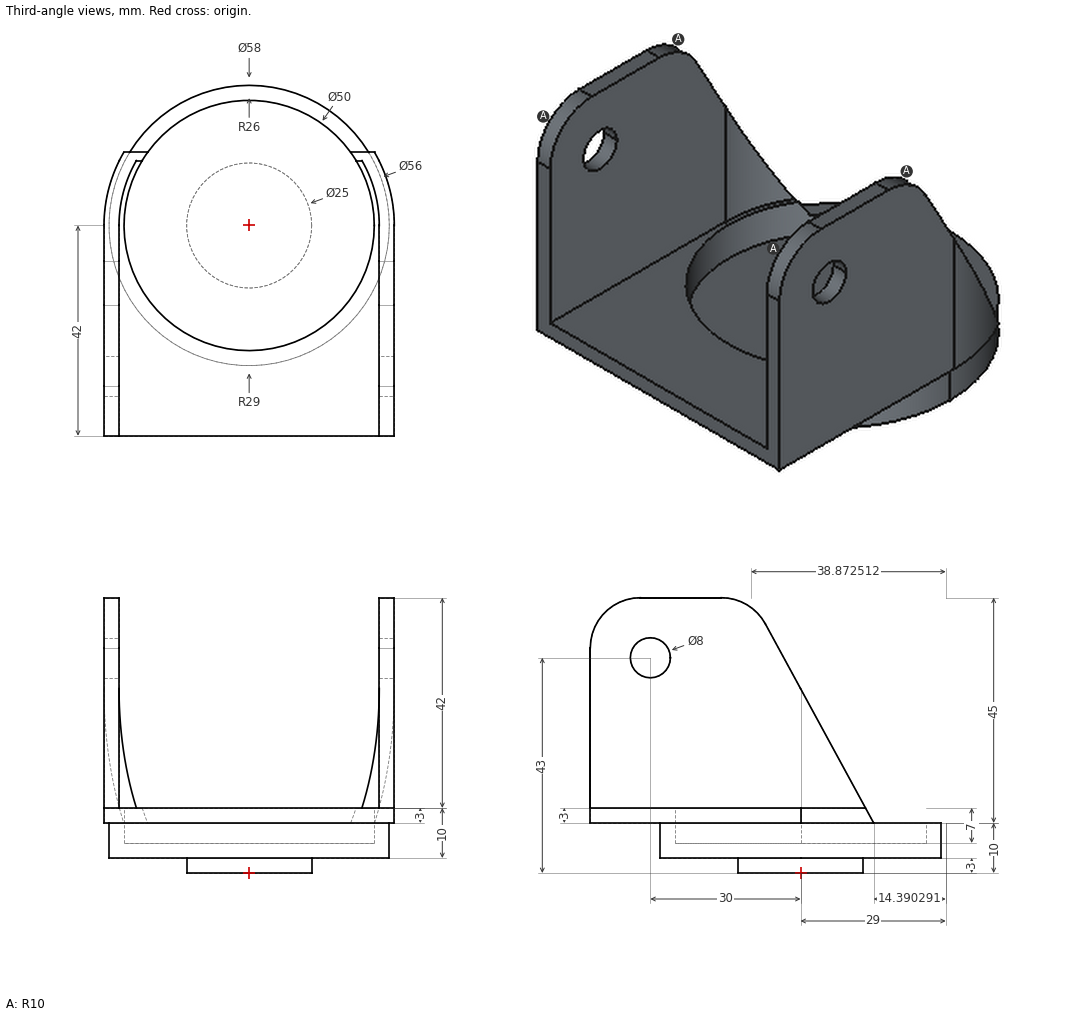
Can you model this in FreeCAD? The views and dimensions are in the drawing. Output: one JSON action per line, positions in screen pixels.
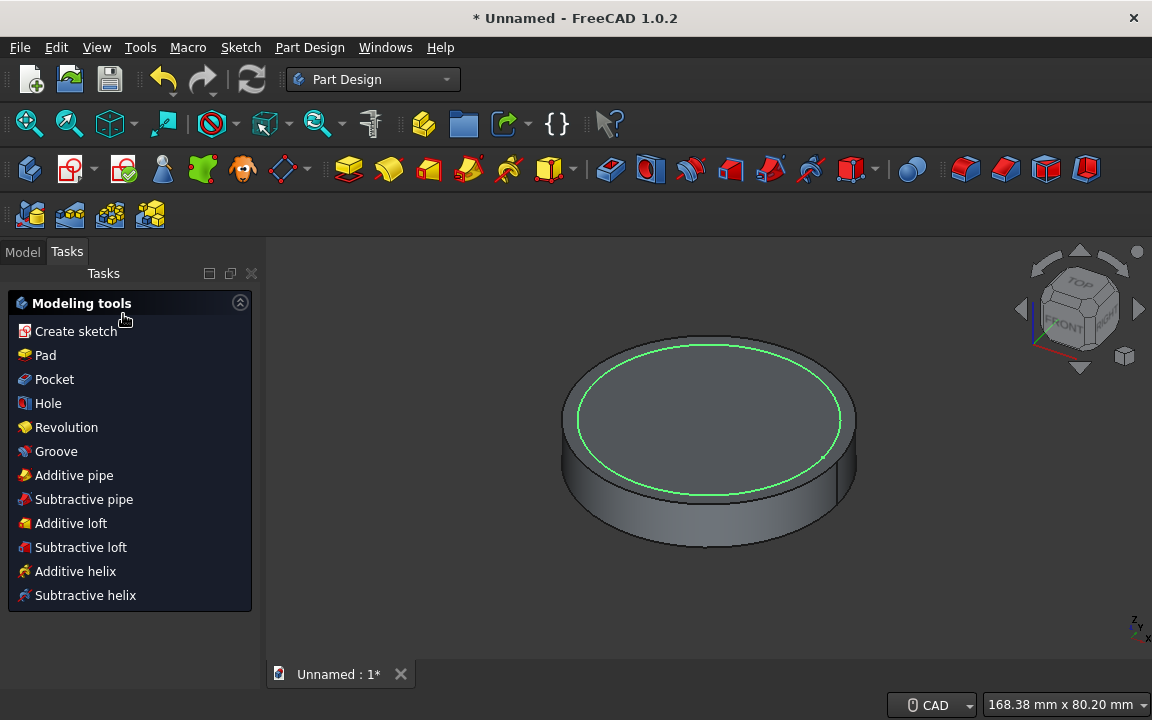
{"action": "left_click", "coordinate": [612, 170]}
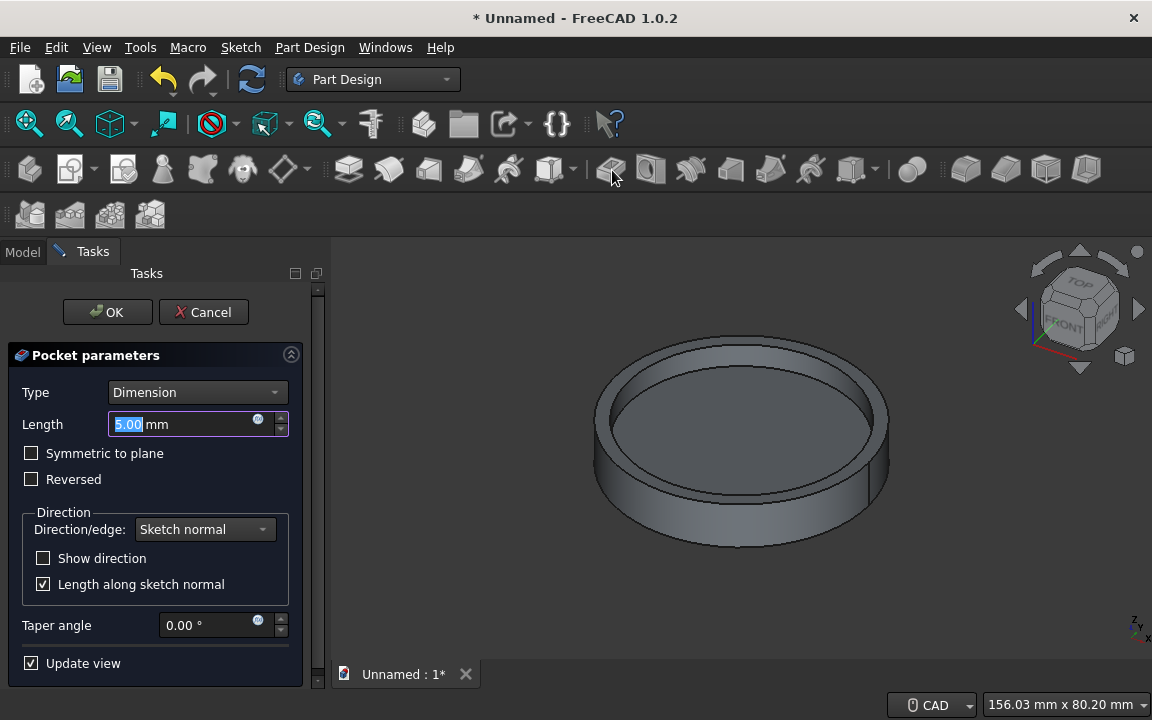
{"action": "type", "text": "7"}
{"action": "key", "text": "Tab"}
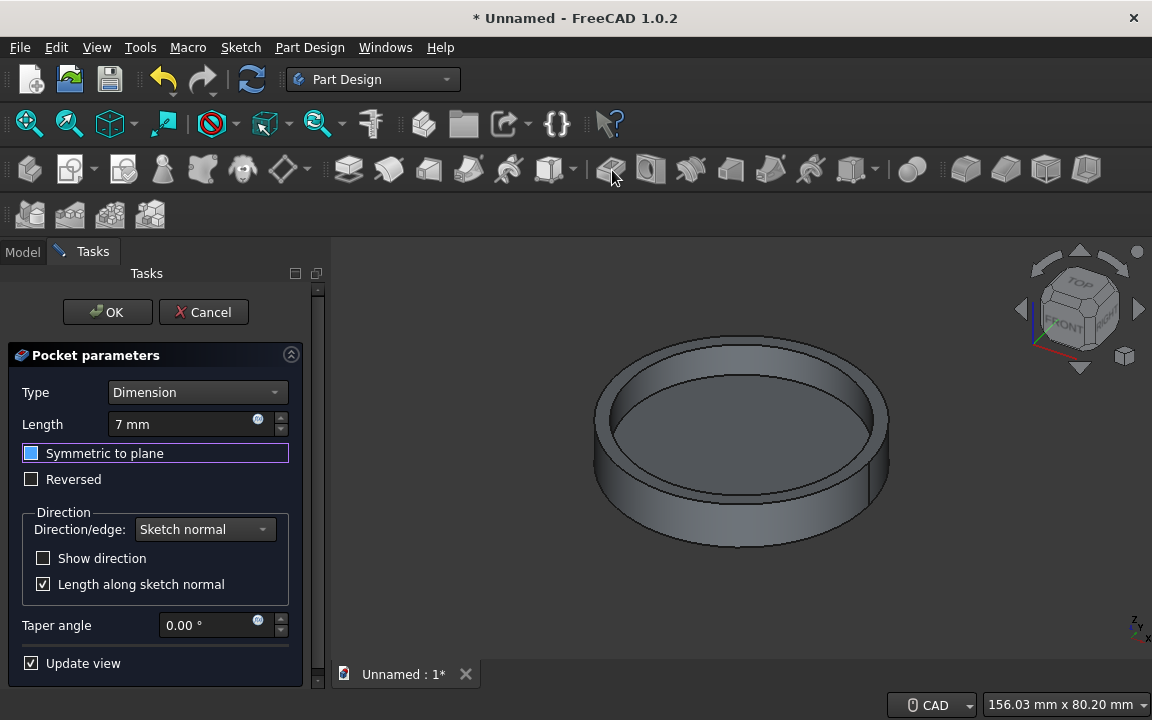
{"action": "left_click", "coordinate": [108, 312]}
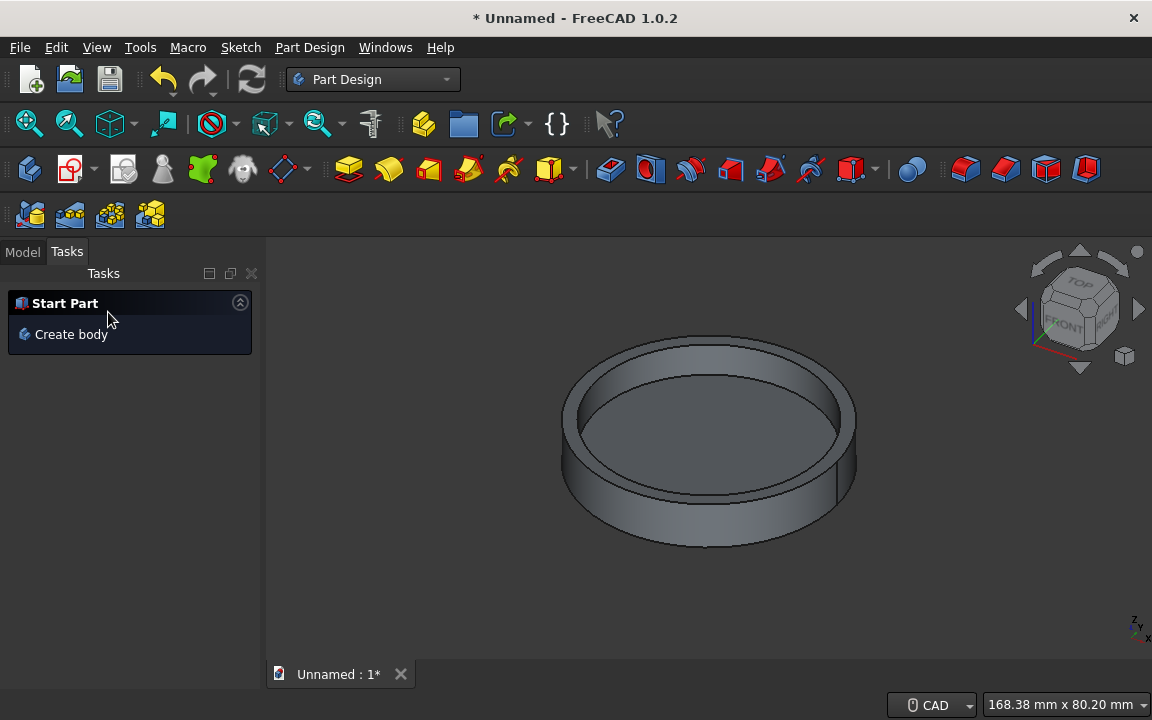
{"action": "scroll", "coordinate": [809, 368], "scroll_direction": "up", "scroll_amount": 11}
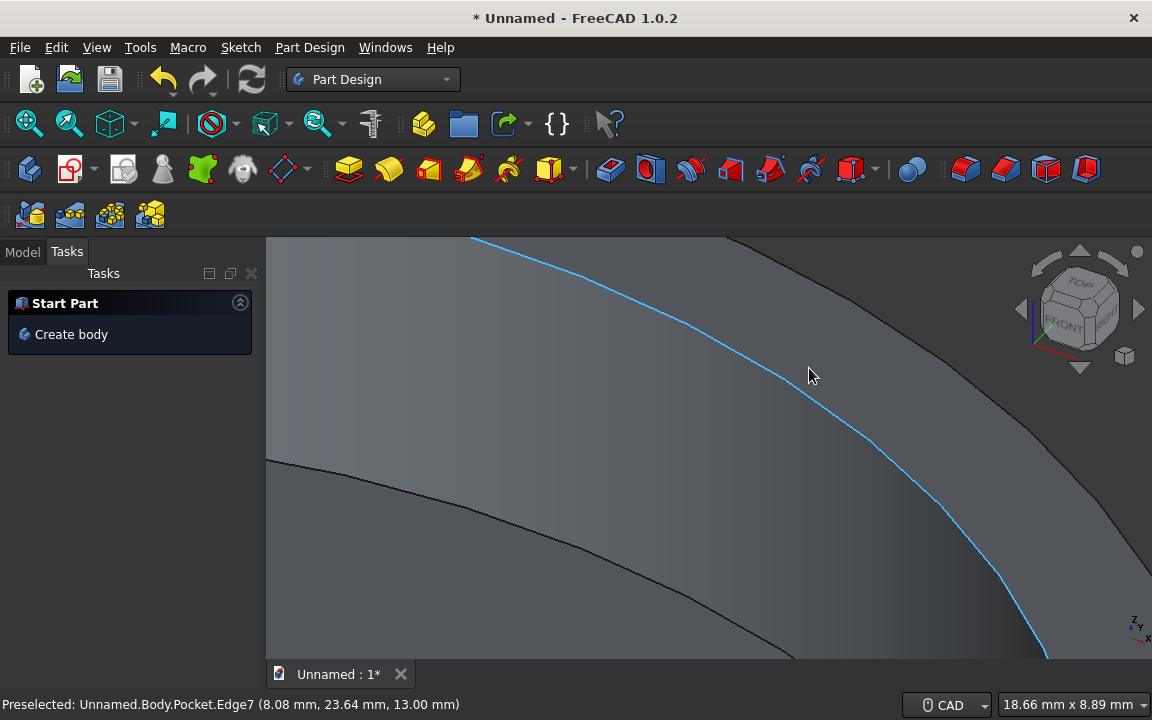
{"action": "left_click", "coordinate": [800, 376]}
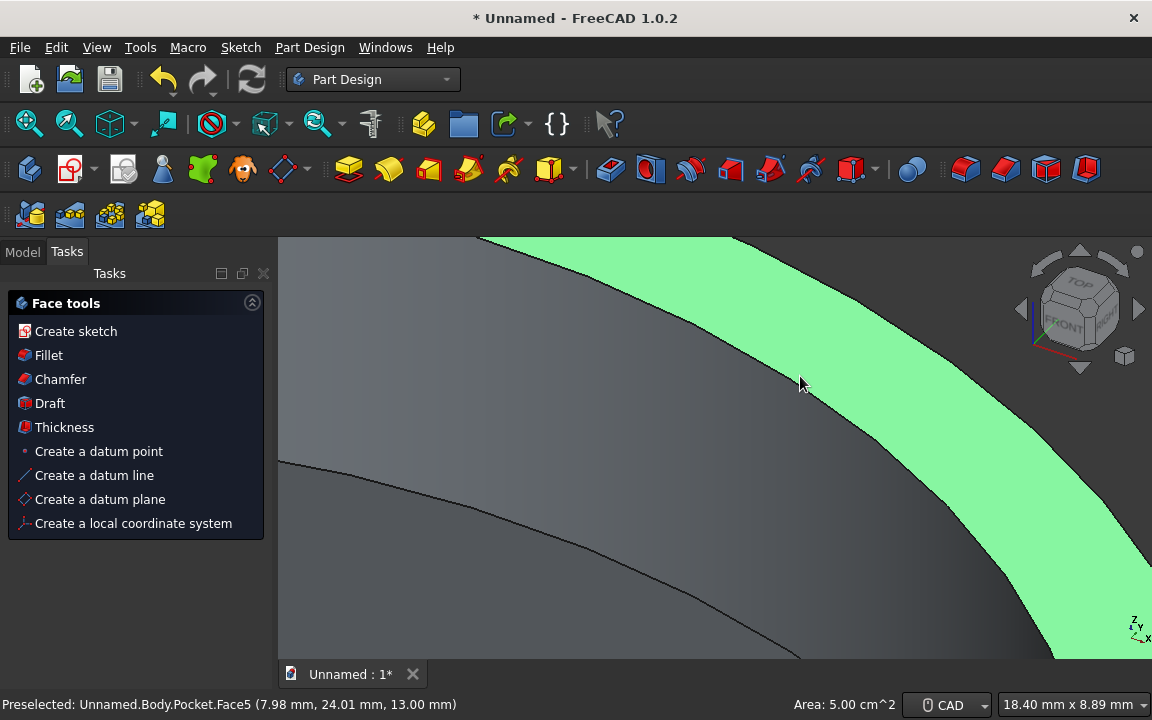
{"action": "left_click", "coordinate": [70, 170]}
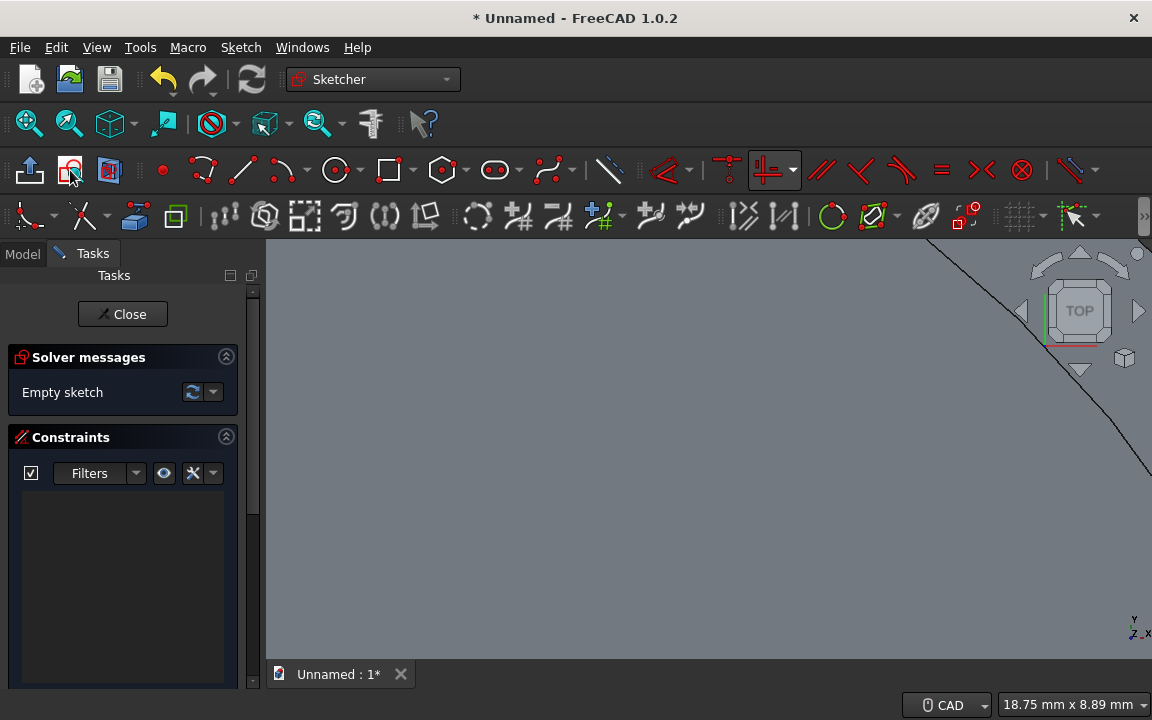
{"action": "scroll", "coordinate": [685, 377], "scroll_direction": "down", "scroll_amount": 12}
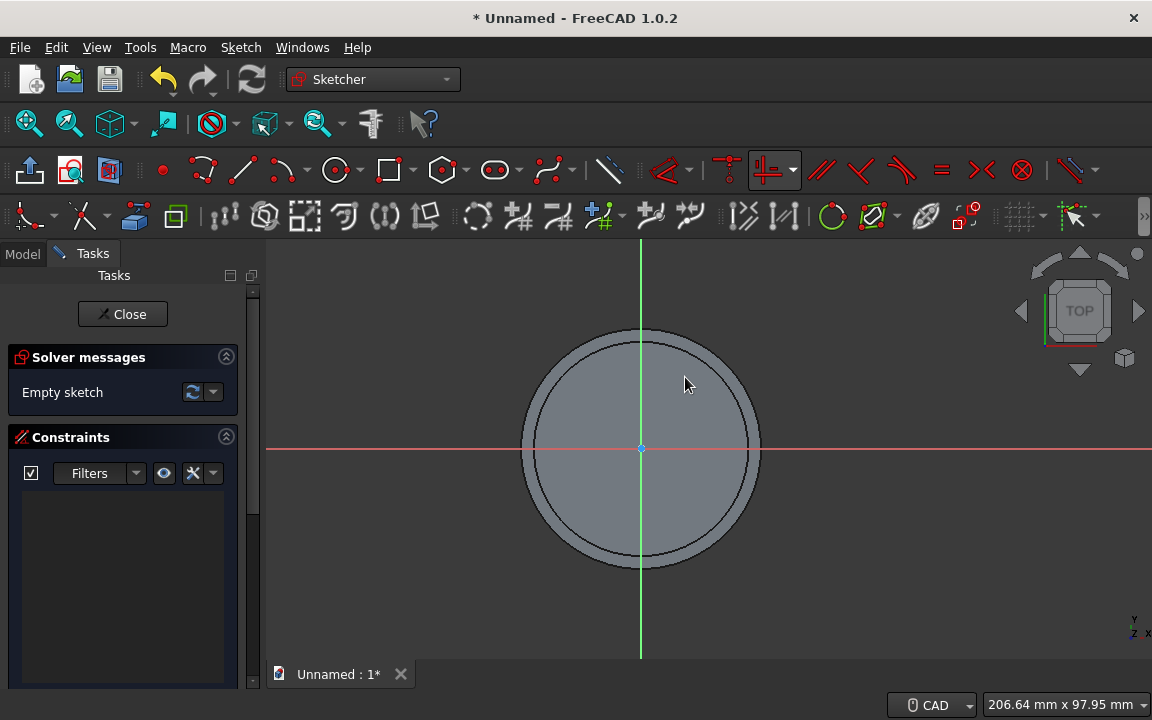
{"action": "left_click", "coordinate": [336, 170]}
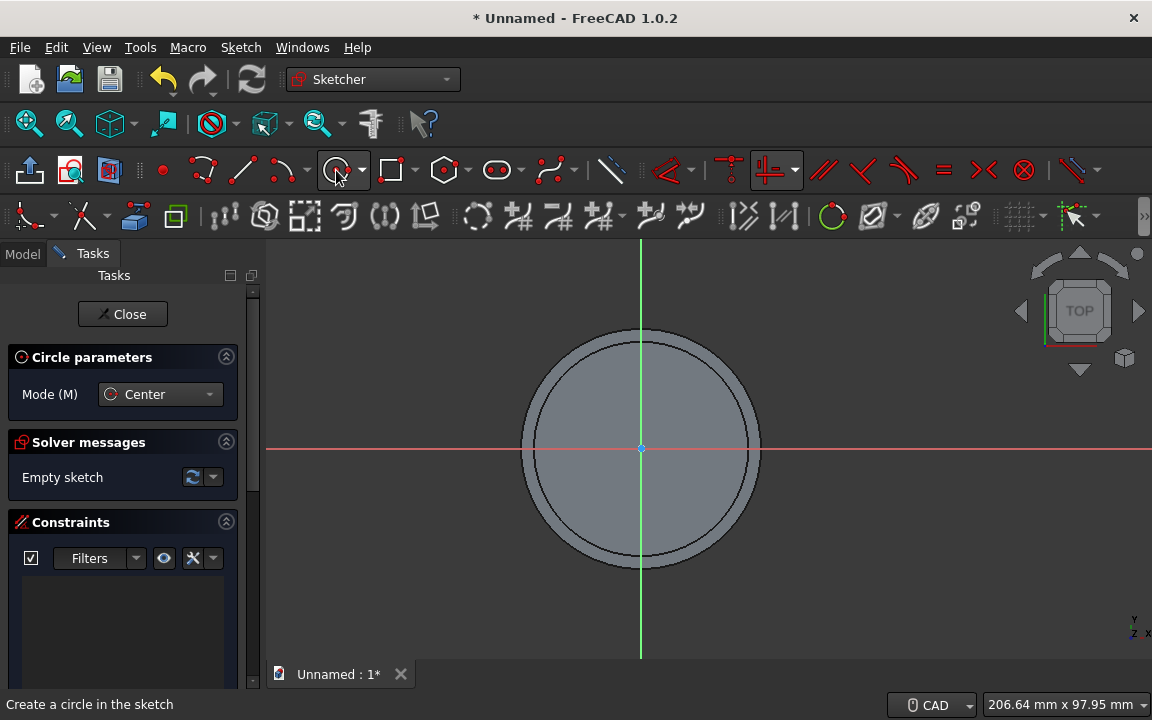
{"action": "left_click", "coordinate": [641, 449]}
{"action": "left_click", "coordinate": [729, 361]}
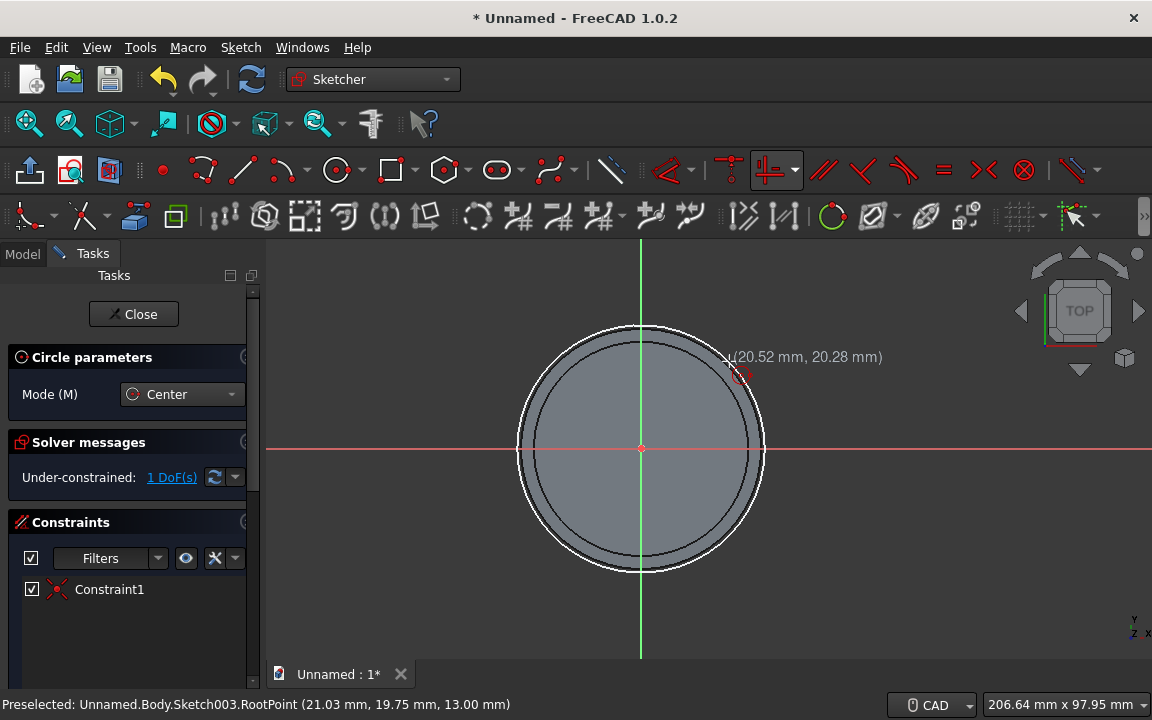
{"action": "left_click", "coordinate": [641, 449]}
{"action": "left_click", "coordinate": [717, 373]}
{"action": "key", "text": "Escape"}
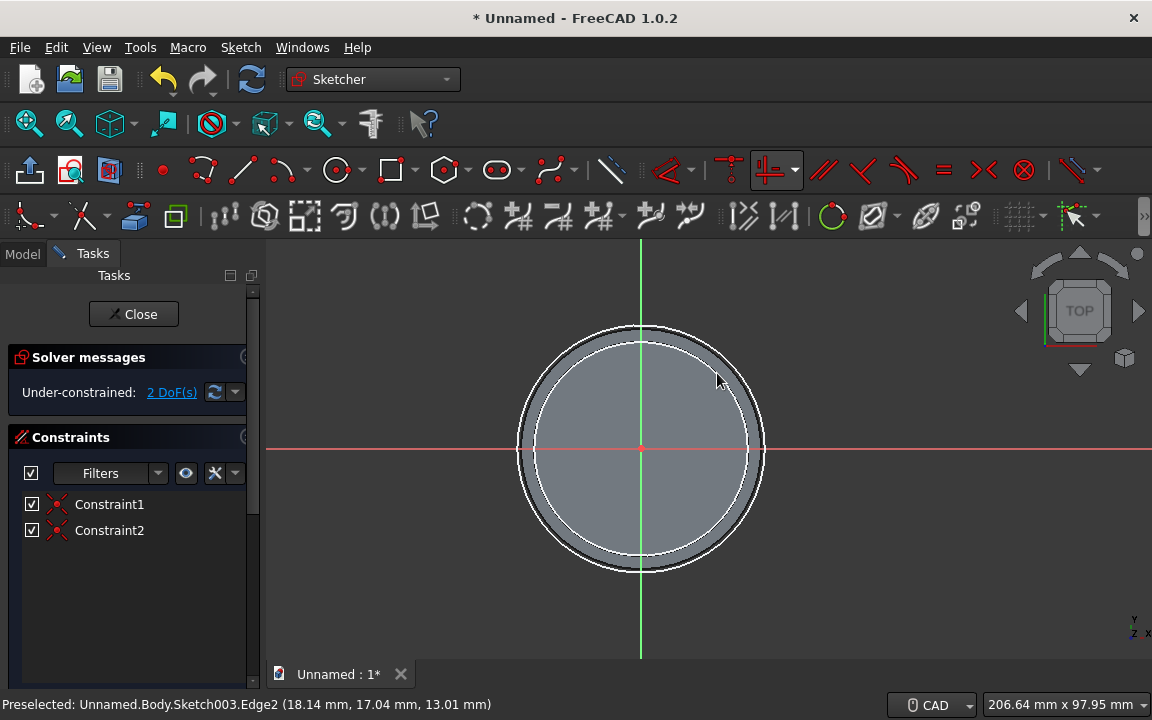
{"action": "left_click", "coordinate": [666, 170]}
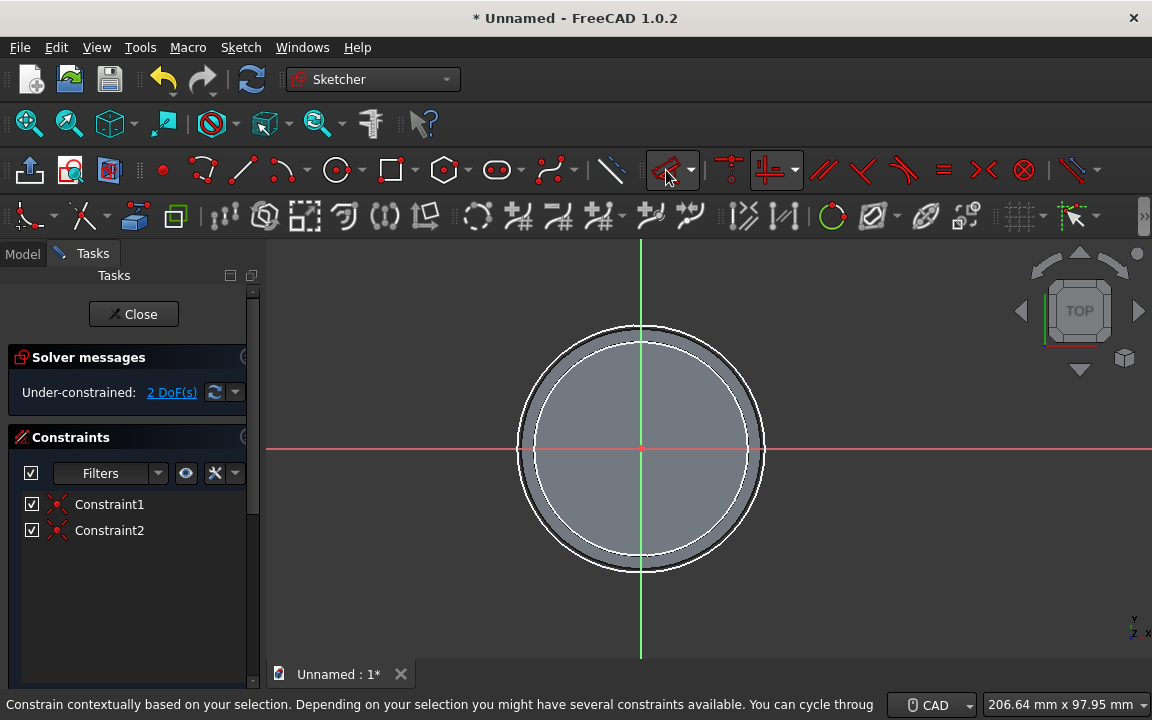
{"action": "left_click", "coordinate": [728, 361]}
{"action": "left_click", "coordinate": [750, 338]}